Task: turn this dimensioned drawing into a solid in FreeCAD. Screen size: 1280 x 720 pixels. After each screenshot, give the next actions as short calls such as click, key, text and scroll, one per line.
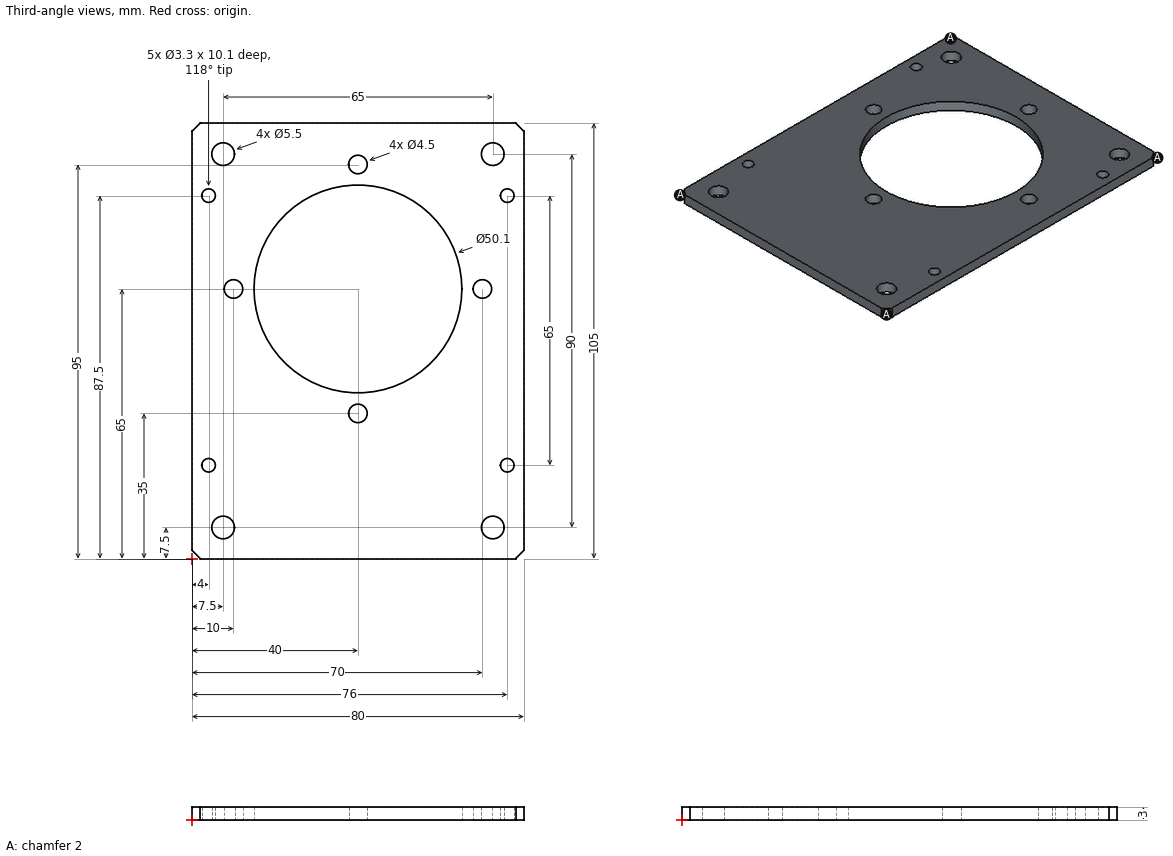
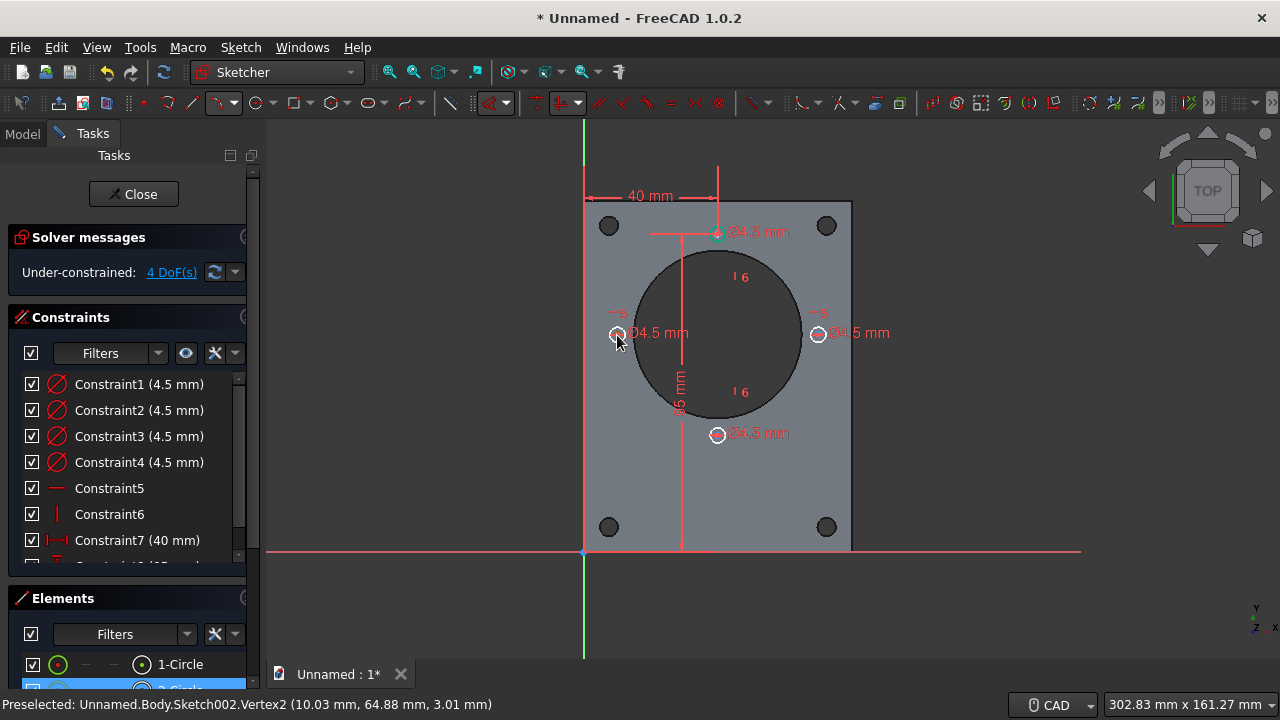
key(l)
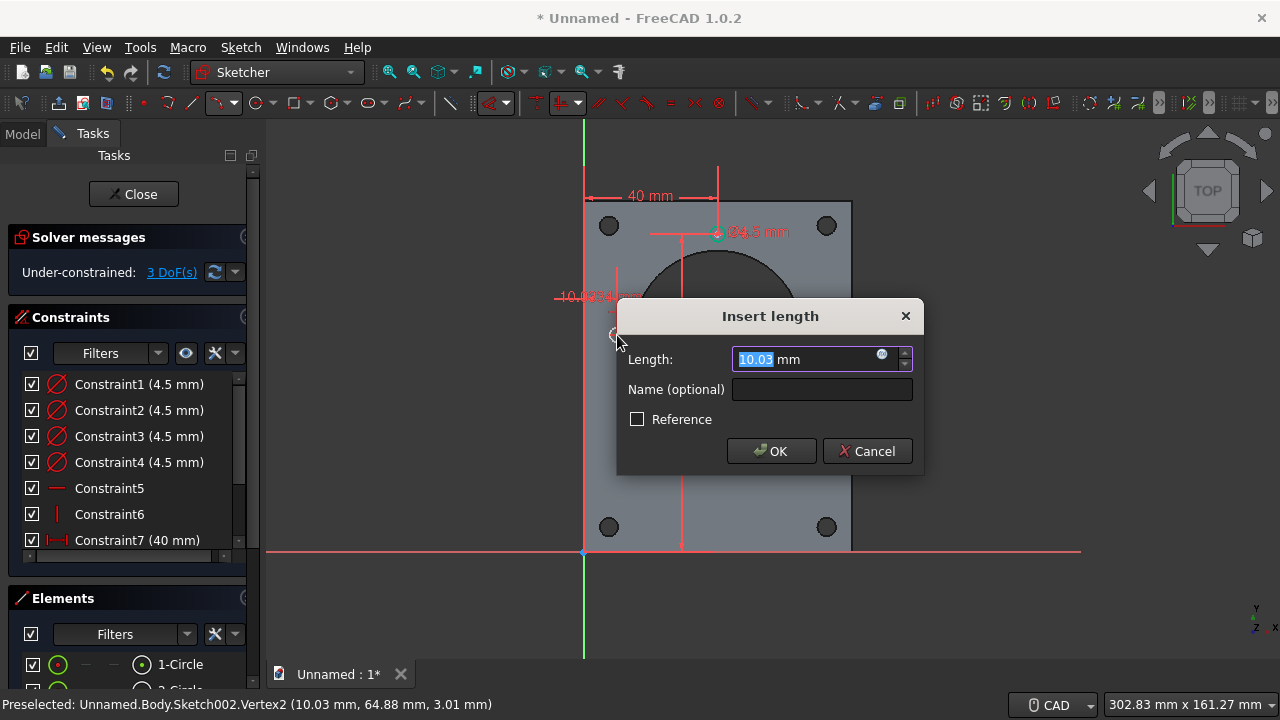
text(10)
key(Return)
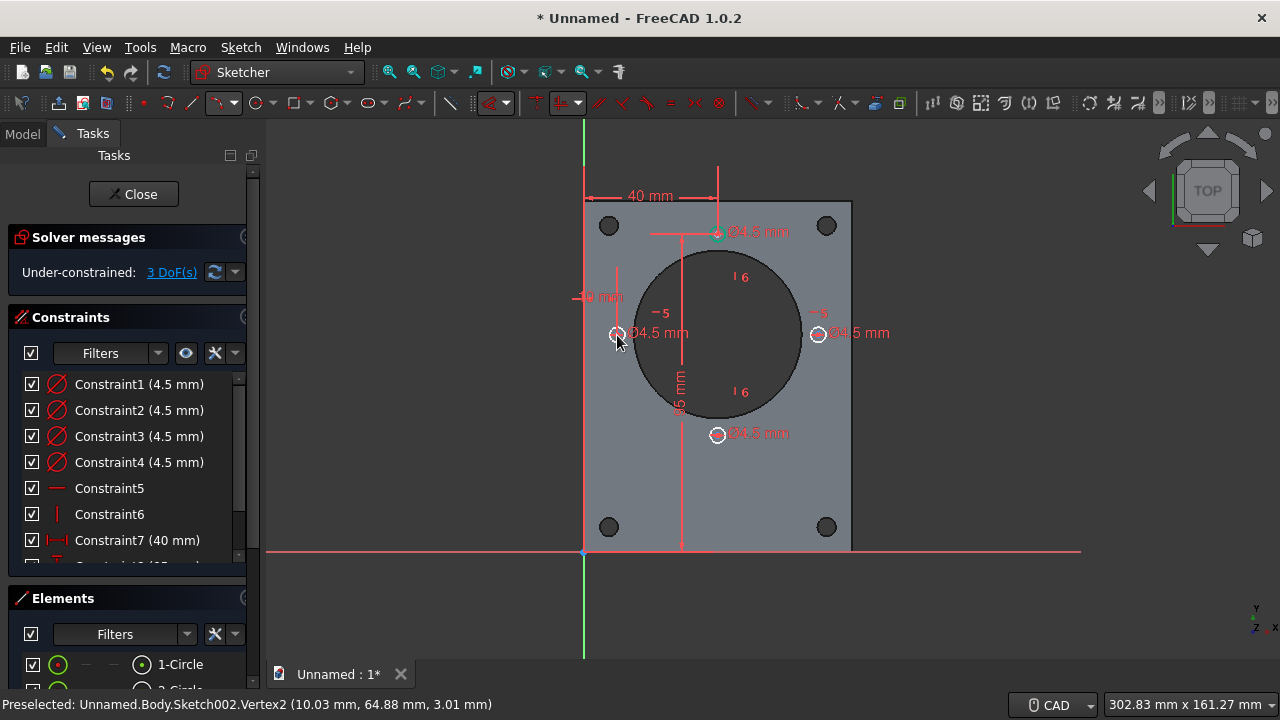
click(617, 335)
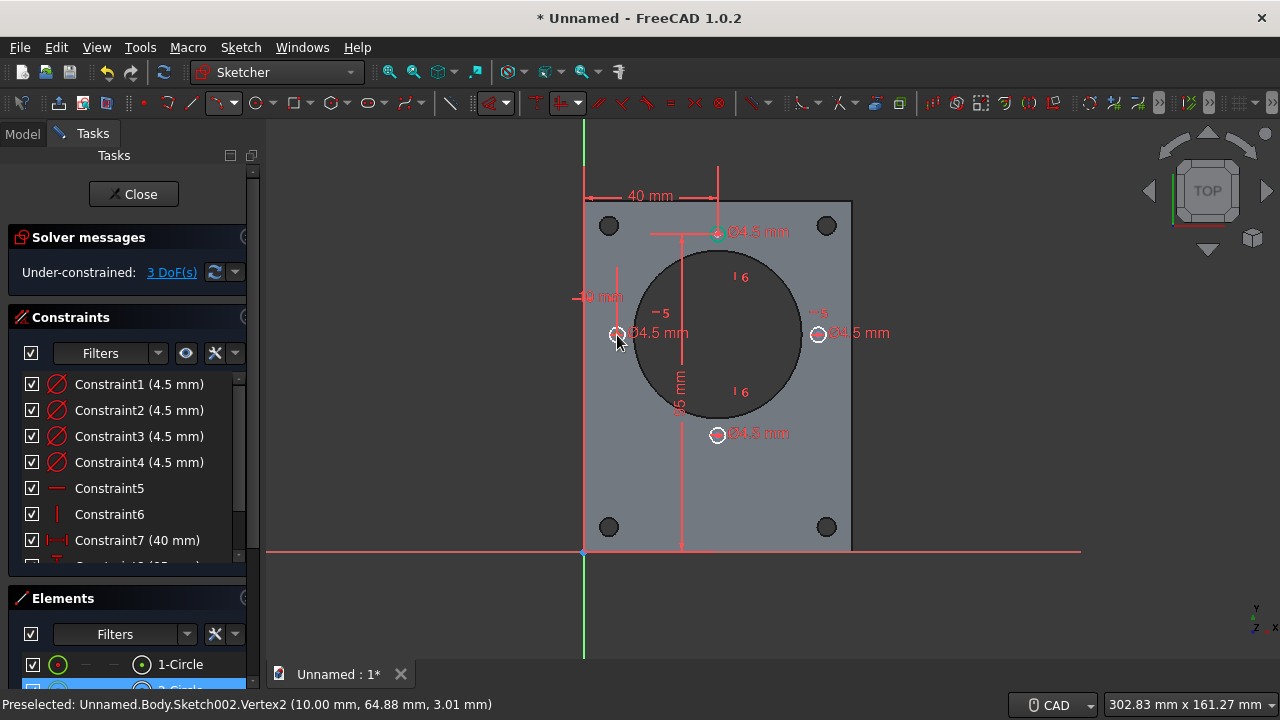
key(i)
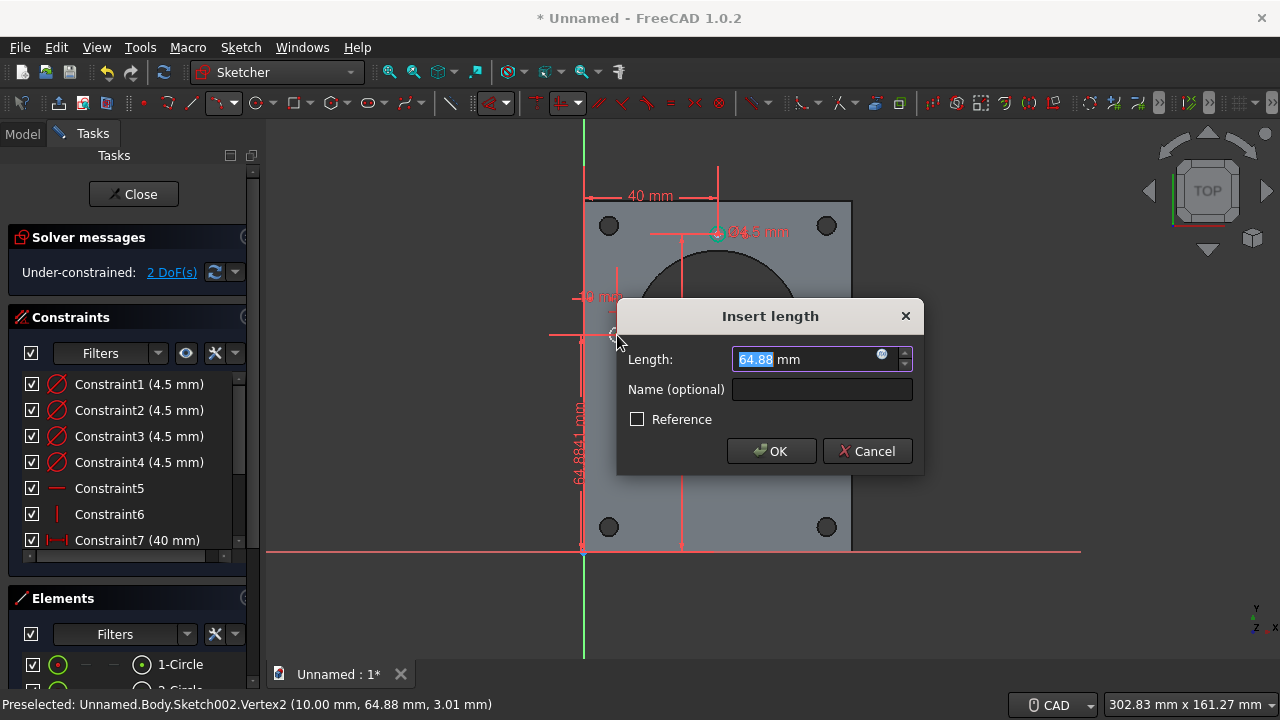
text(65)
key(Return)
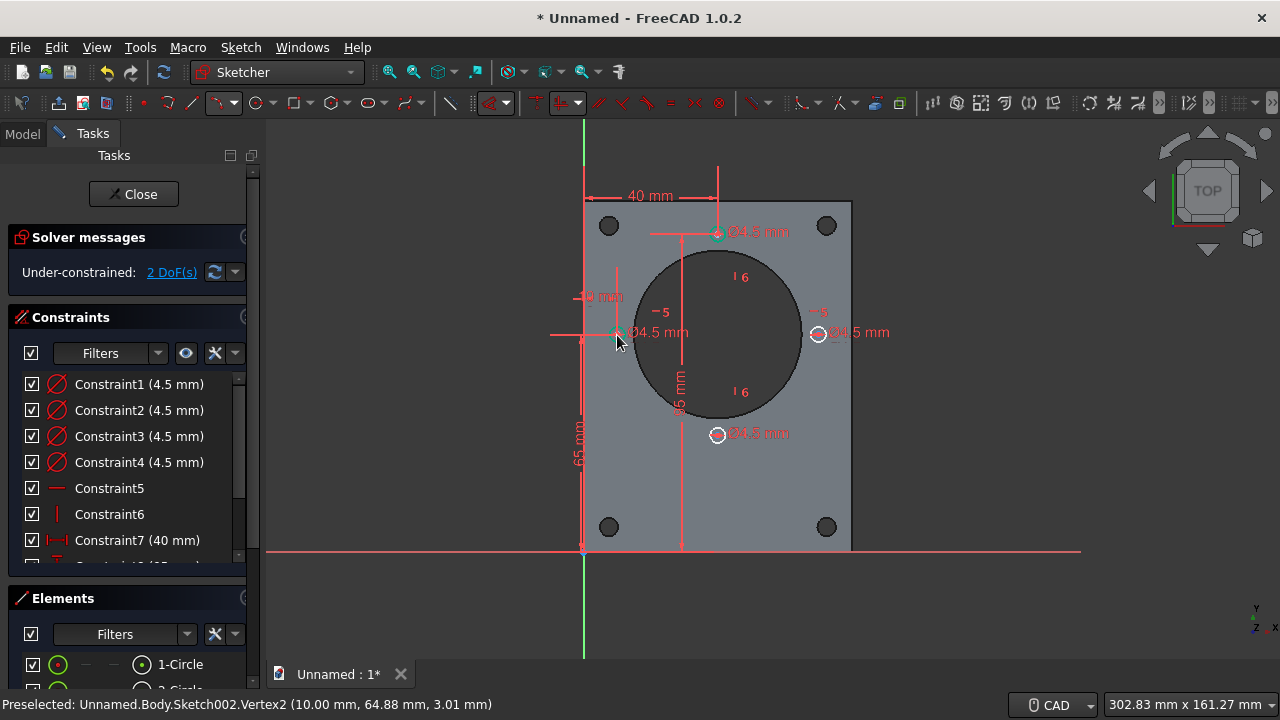
click(818, 335)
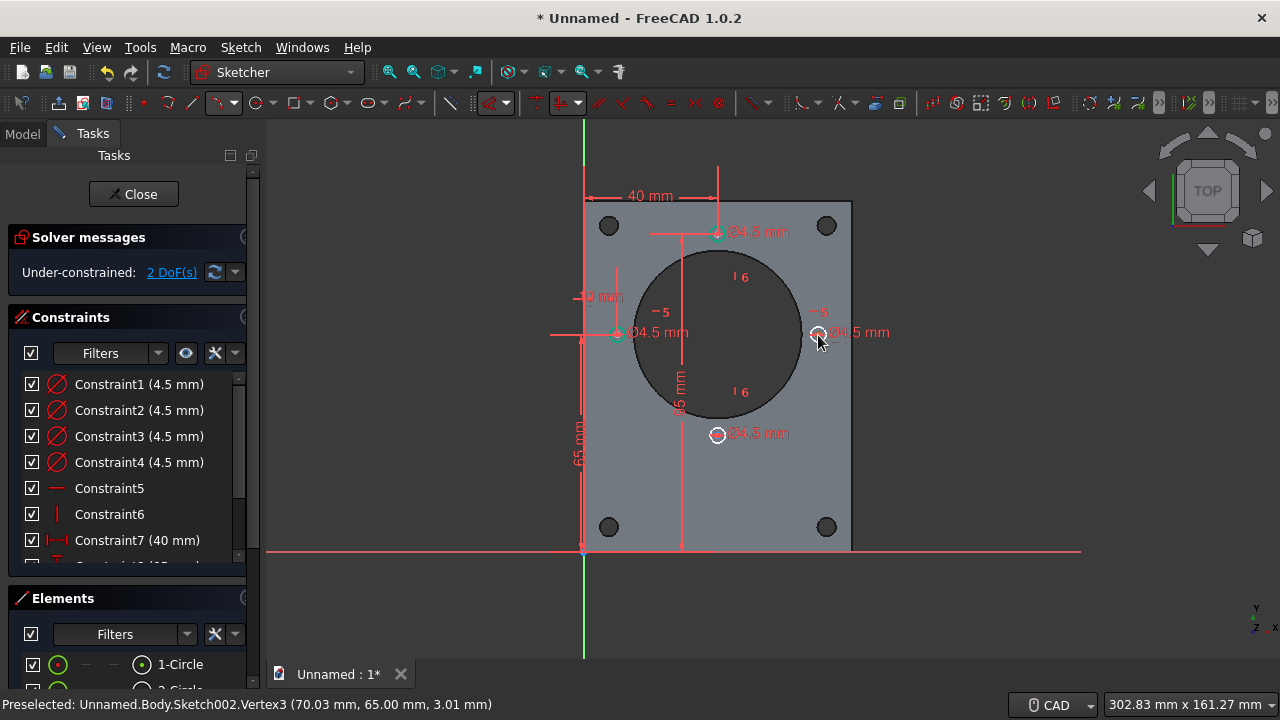
key(l)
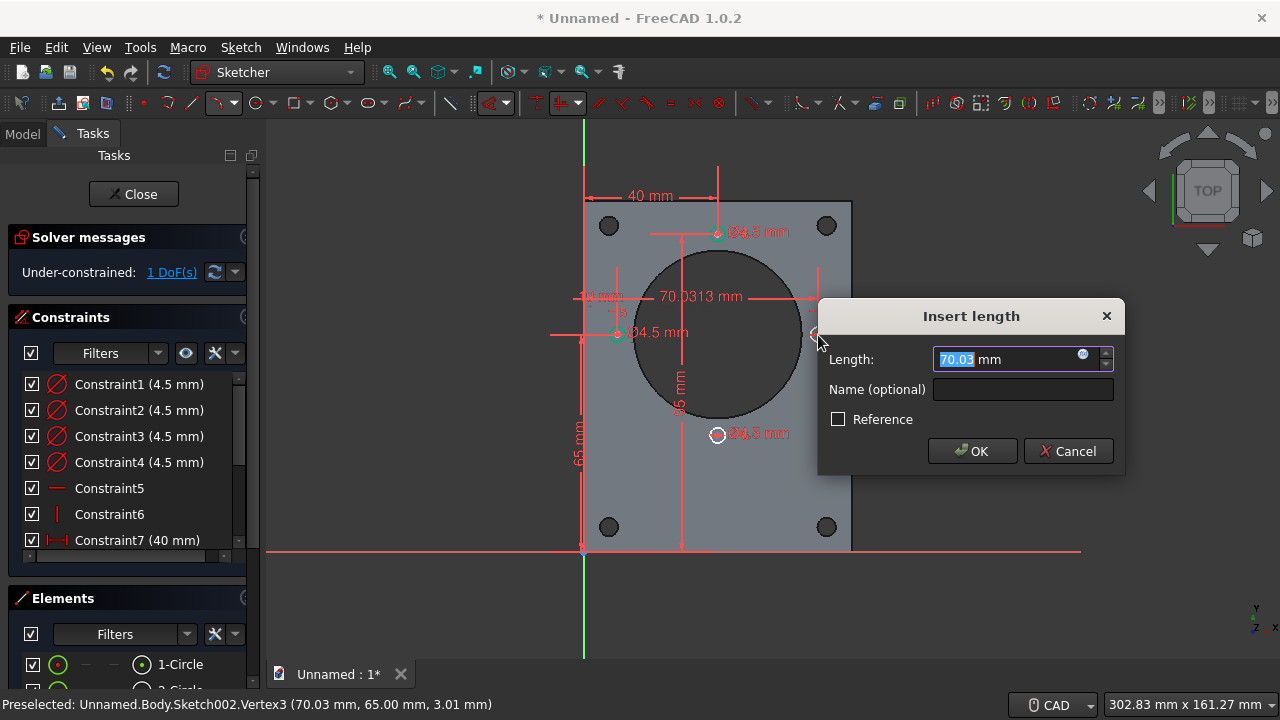
text(70)
key(Return)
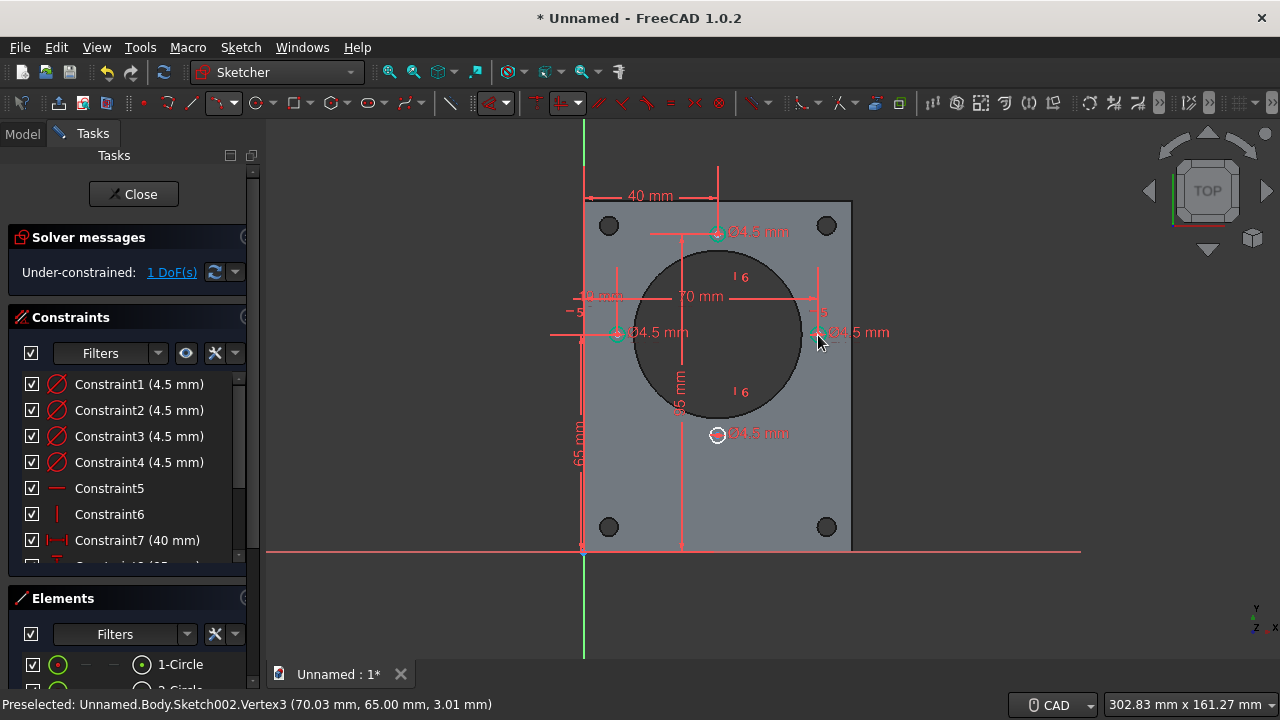
click(718, 435)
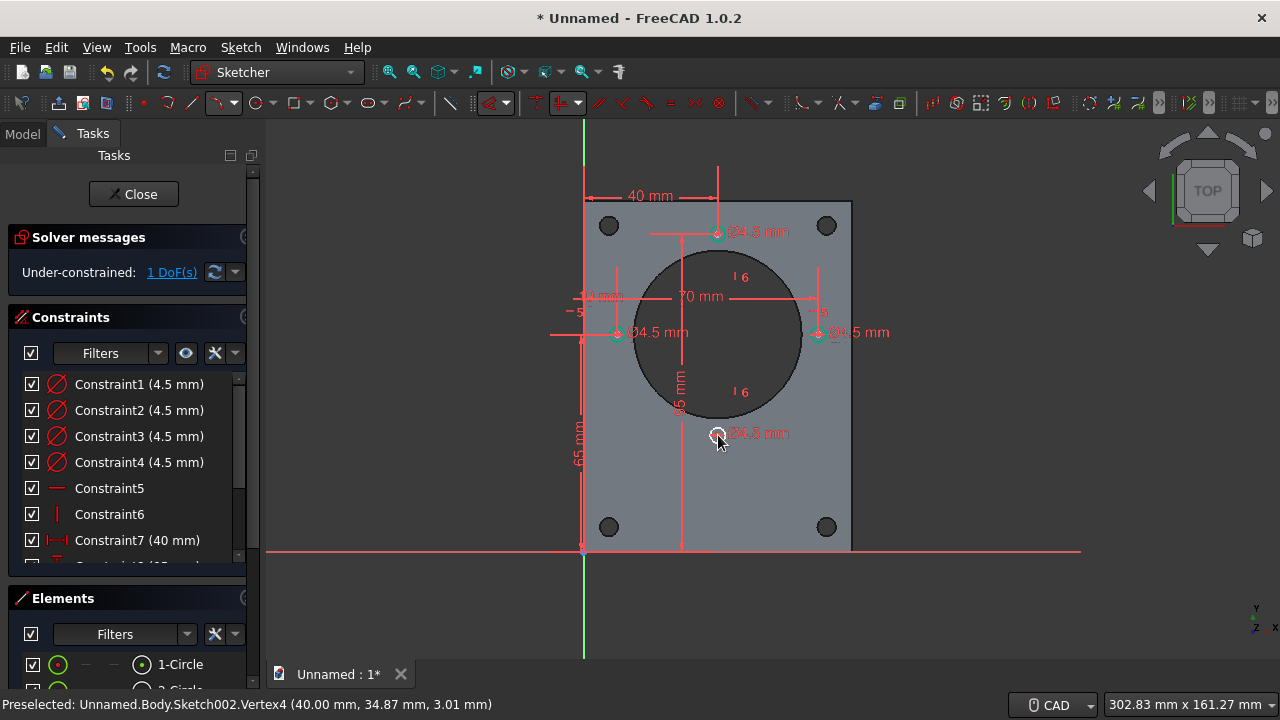
click(508, 104)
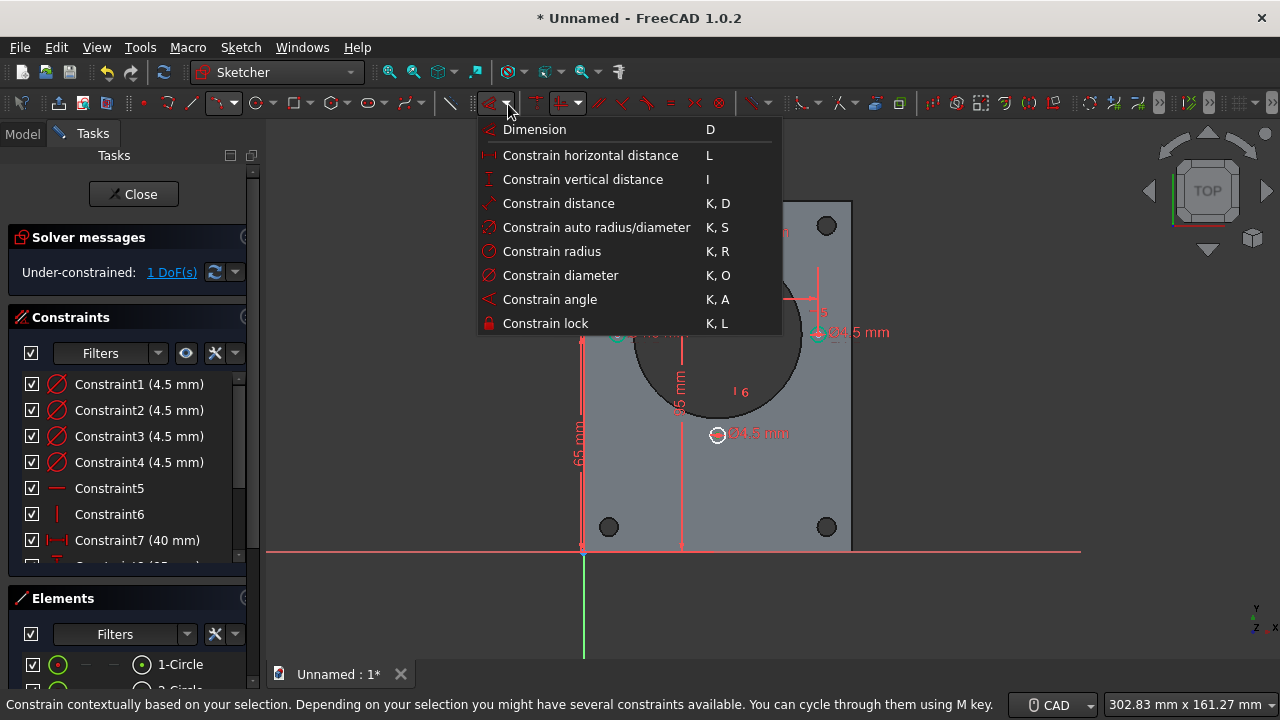
click(630, 179)